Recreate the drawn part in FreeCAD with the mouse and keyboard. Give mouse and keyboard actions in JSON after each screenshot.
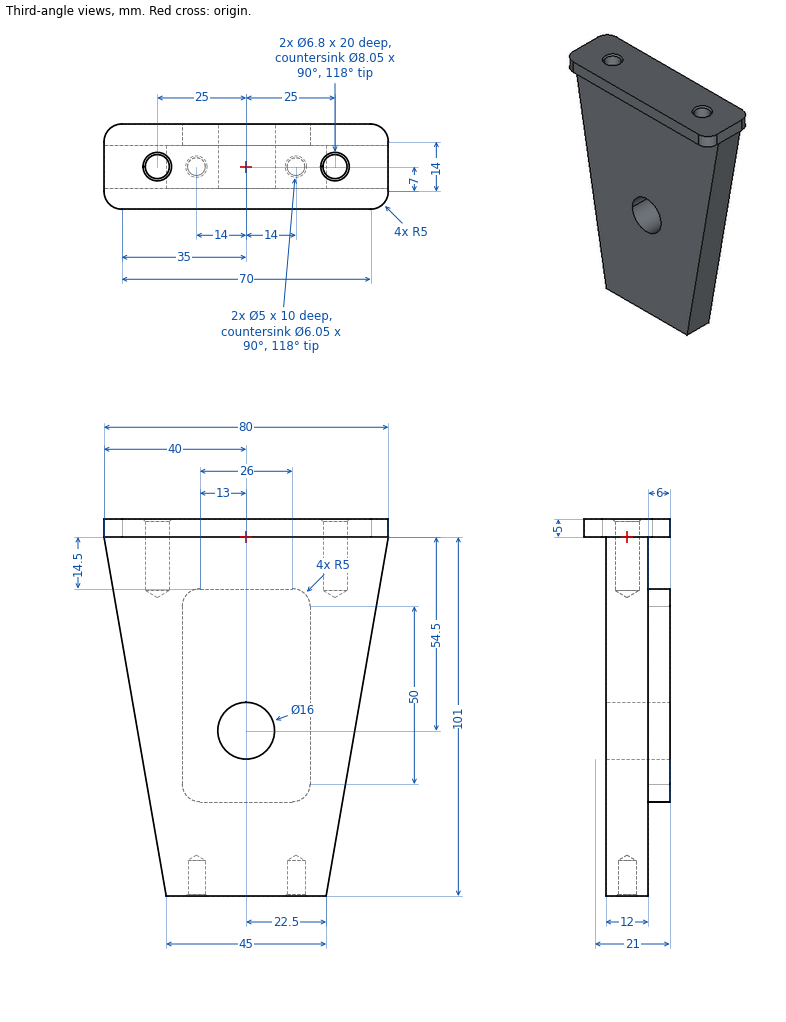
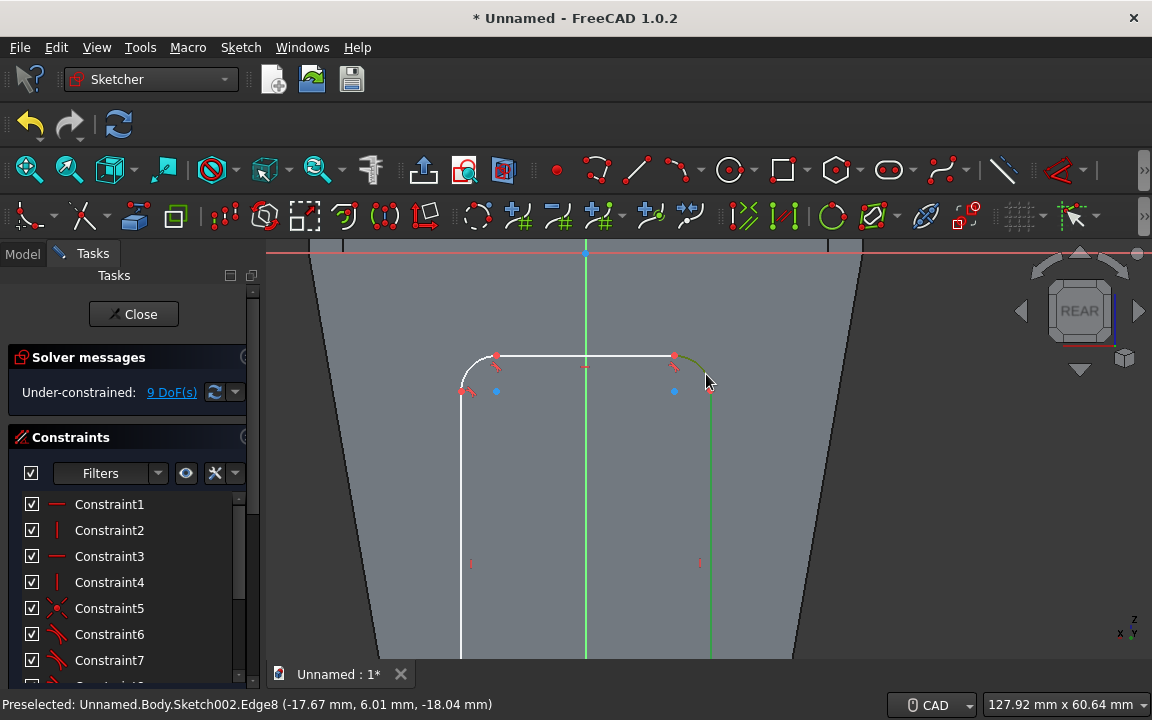
{"action": "key", "text": "t"}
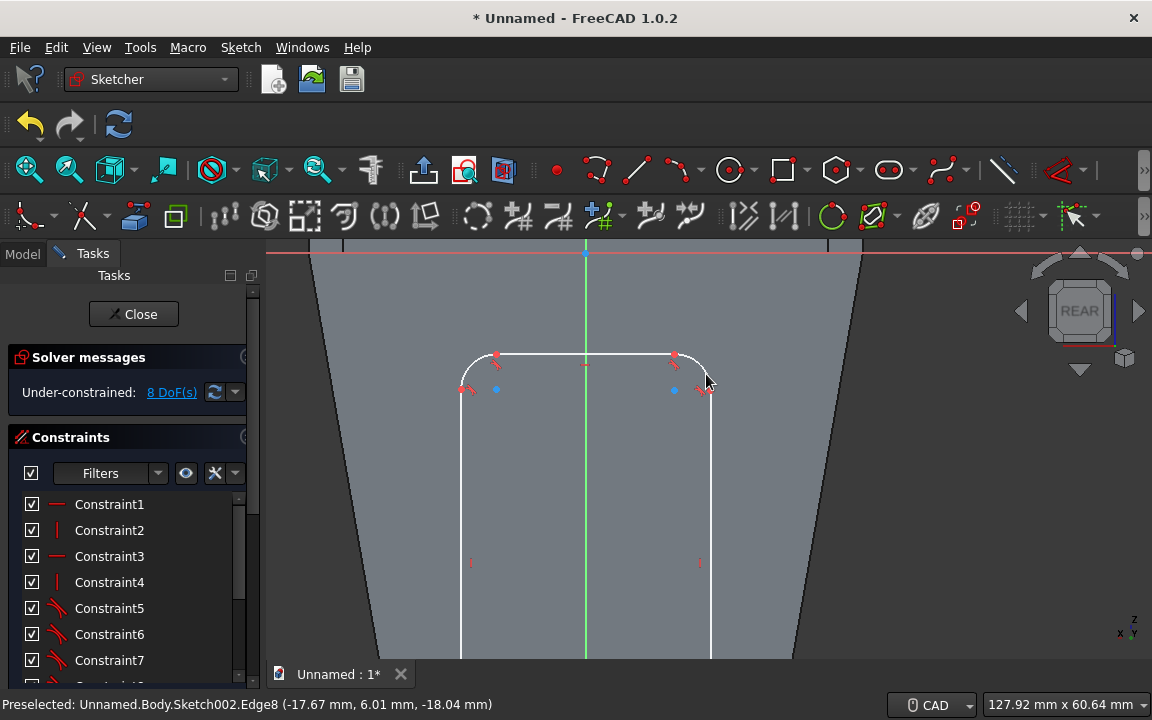
{"action": "left_click", "coordinate": [481, 358]}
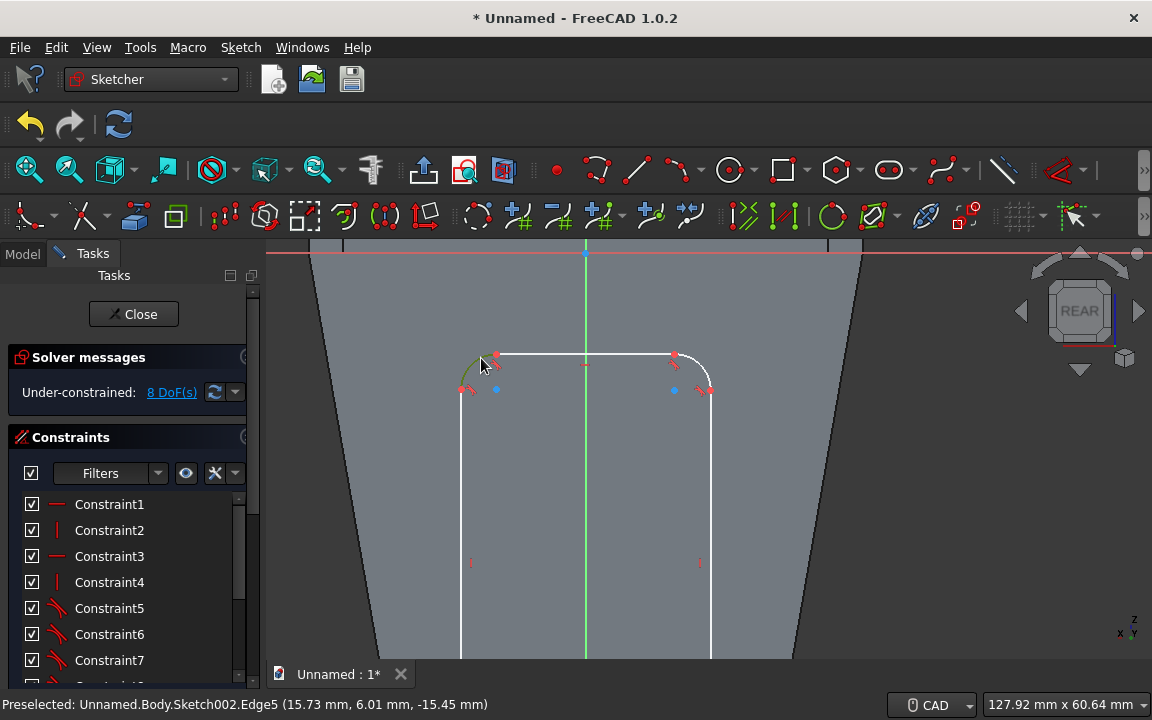
{"action": "scroll", "coordinate": [707, 373], "scroll_direction": "down", "scroll_amount": 3}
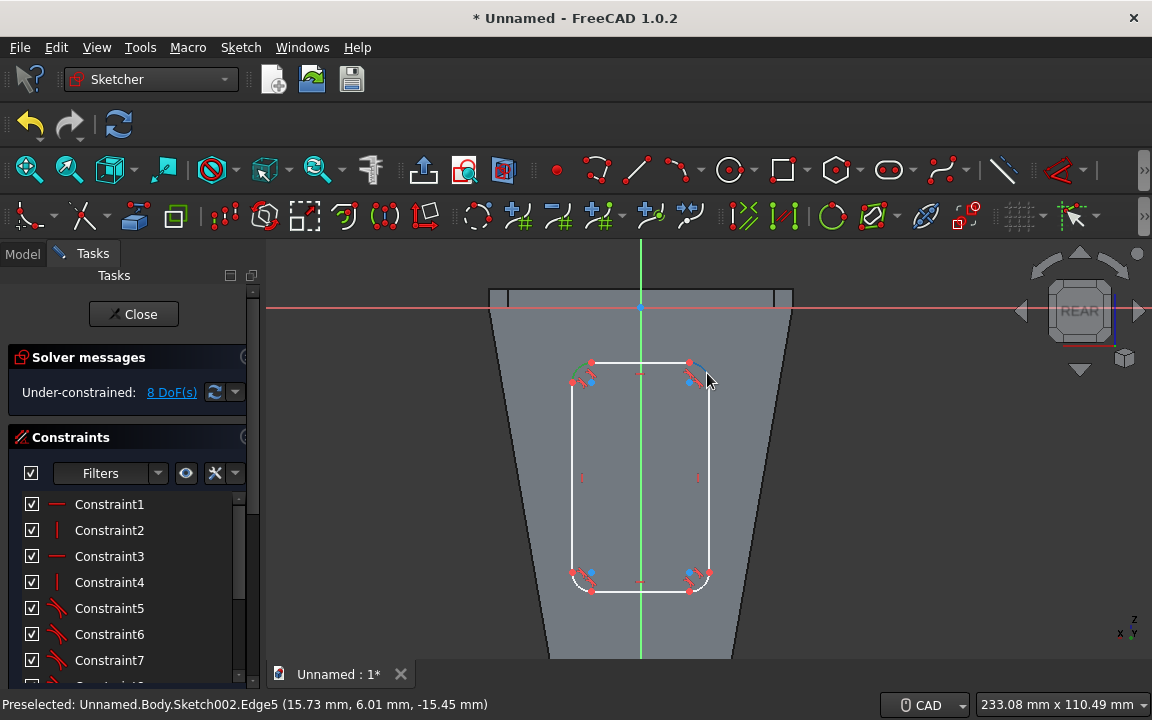
{"action": "scroll", "coordinate": [574, 581], "scroll_direction": "up", "scroll_amount": 3}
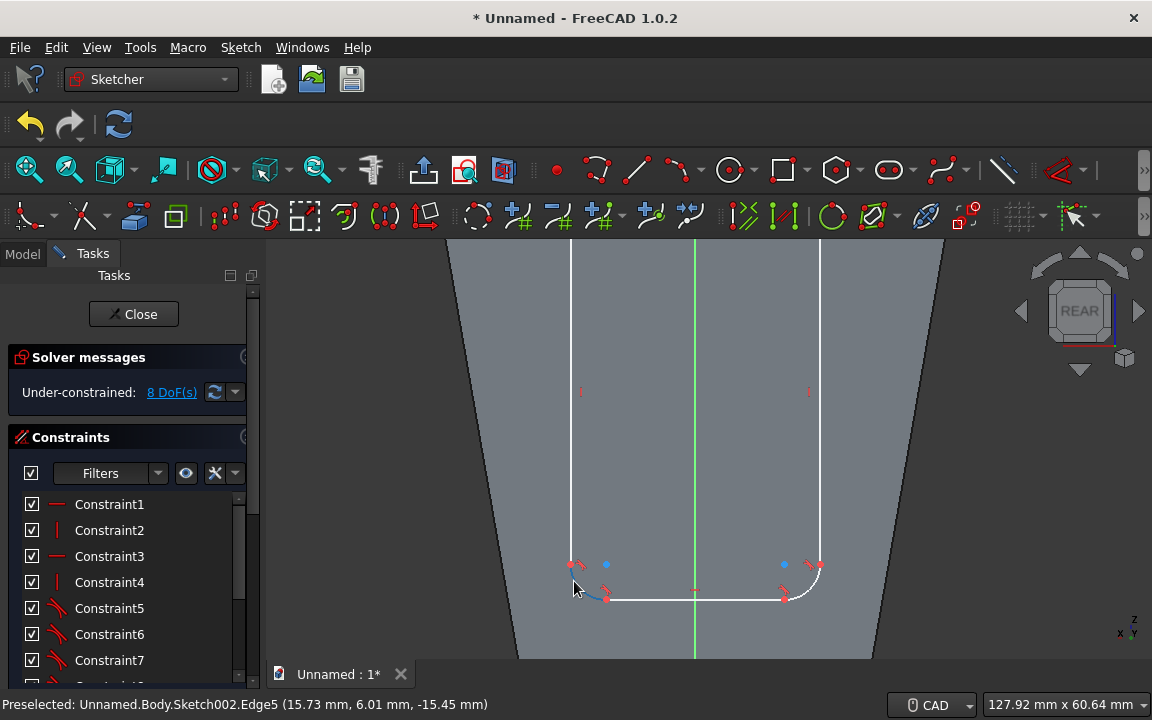
{"action": "left_click", "coordinate": [574, 580]}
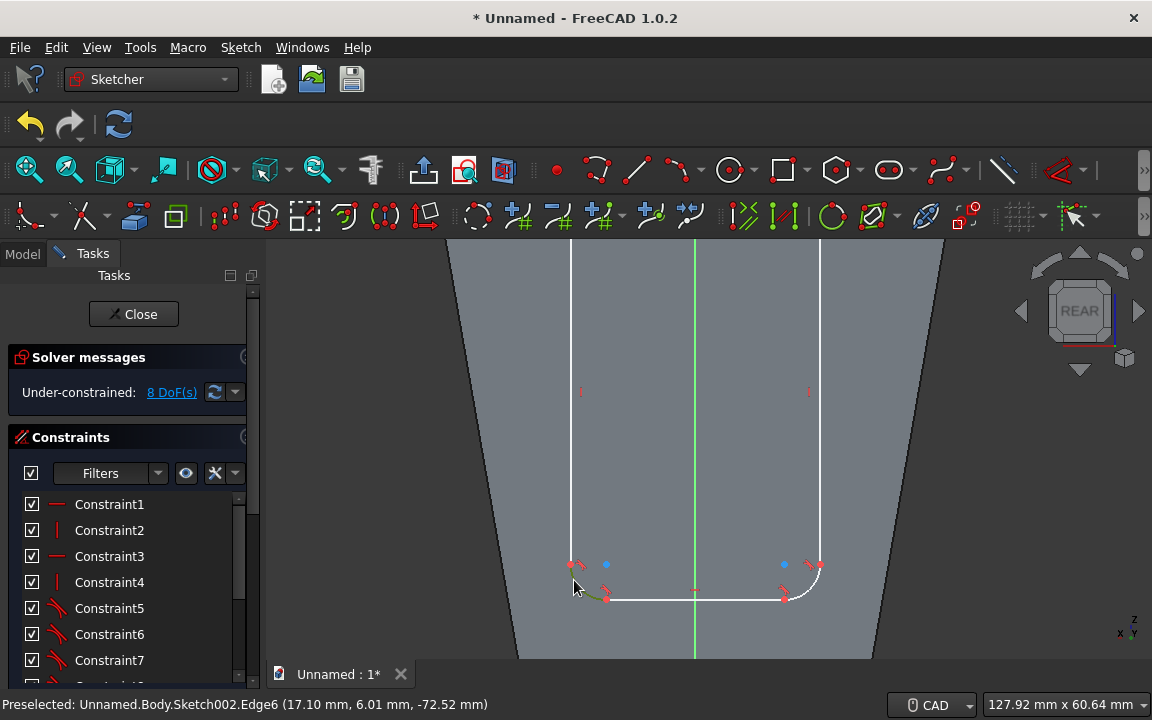
{"action": "left_click", "coordinate": [801, 596]}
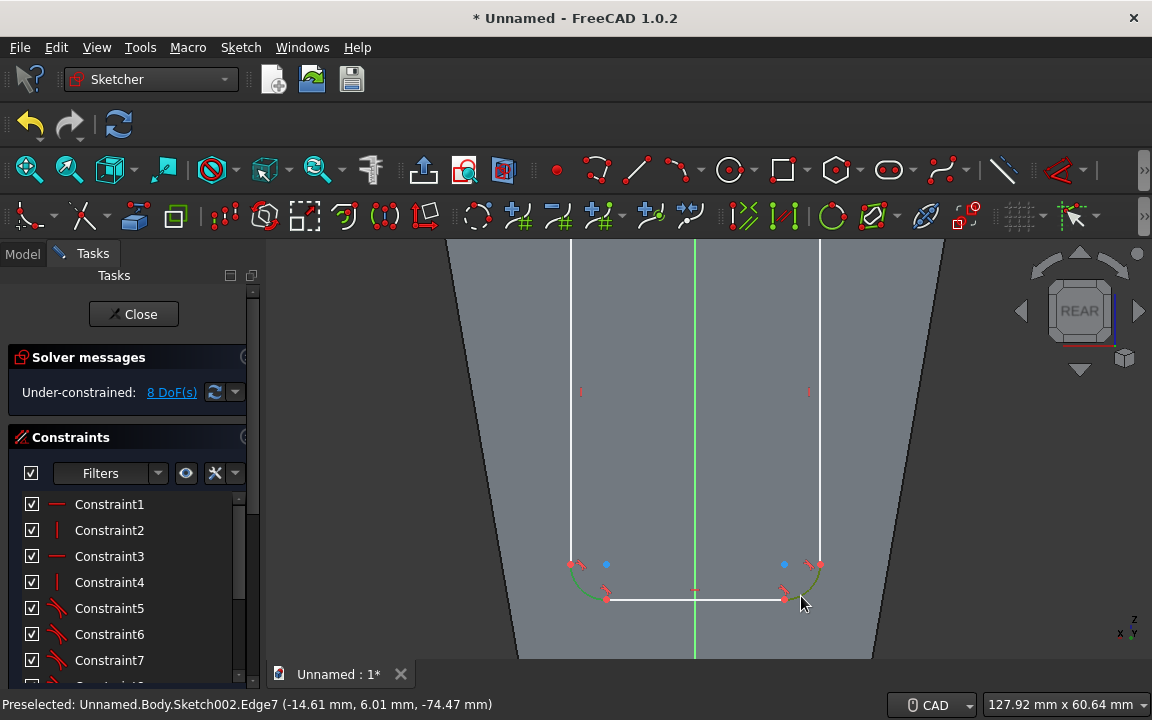
{"action": "scroll", "coordinate": [574, 582], "scroll_direction": "down", "scroll_amount": 3}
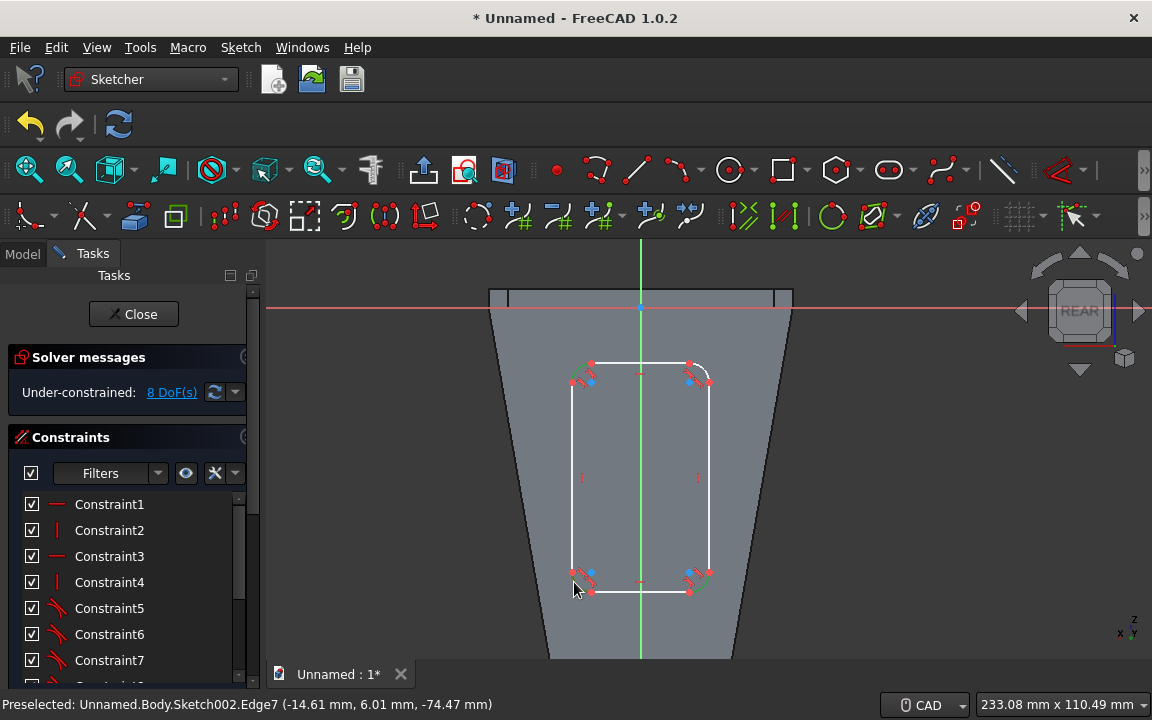
{"action": "scroll", "coordinate": [707, 374], "scroll_direction": "up", "scroll_amount": 3}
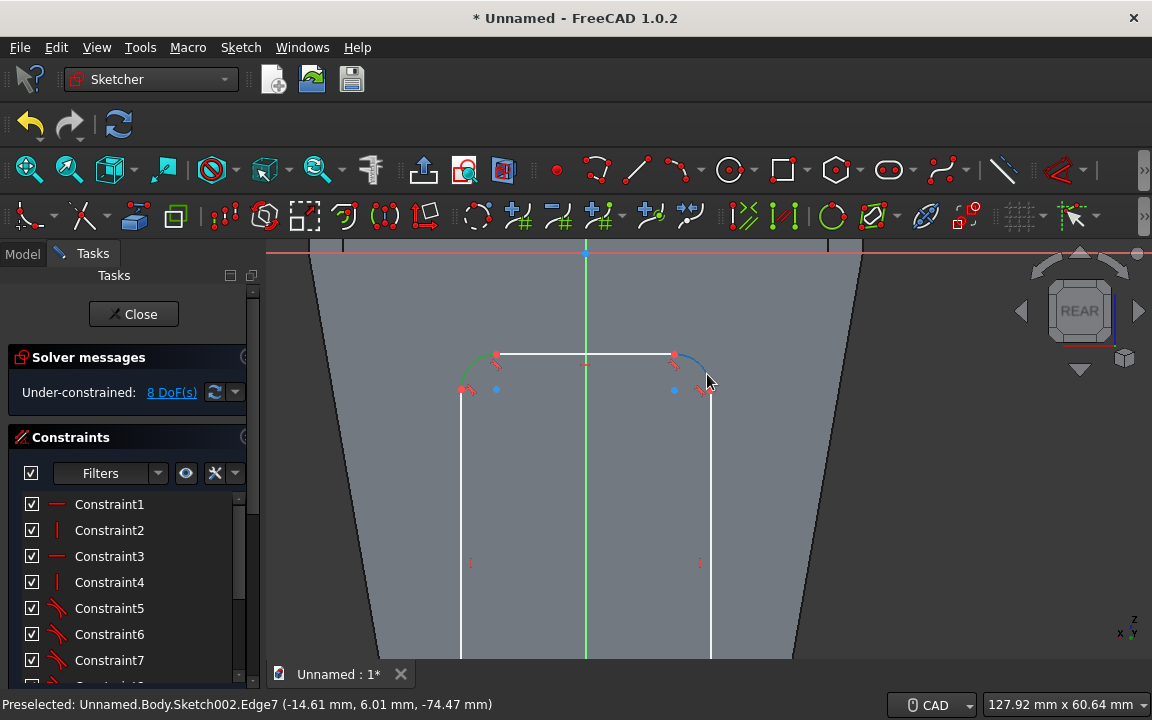
{"action": "left_click", "coordinate": [707, 374]}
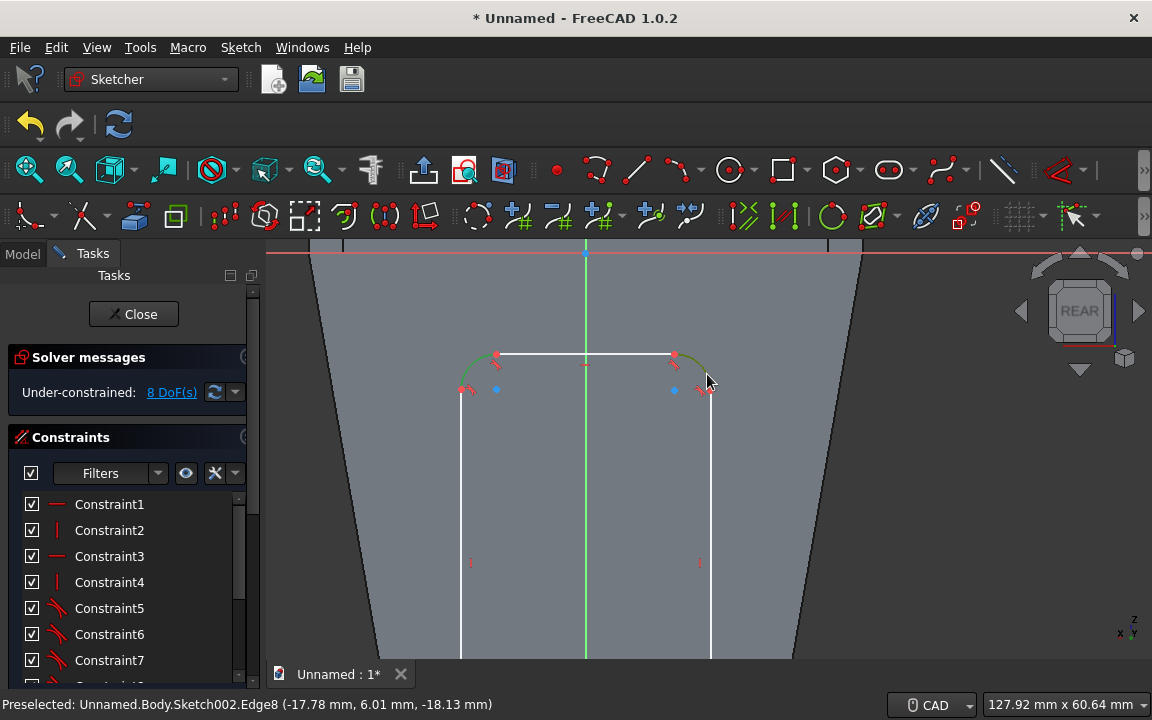
{"action": "key", "text": "e"}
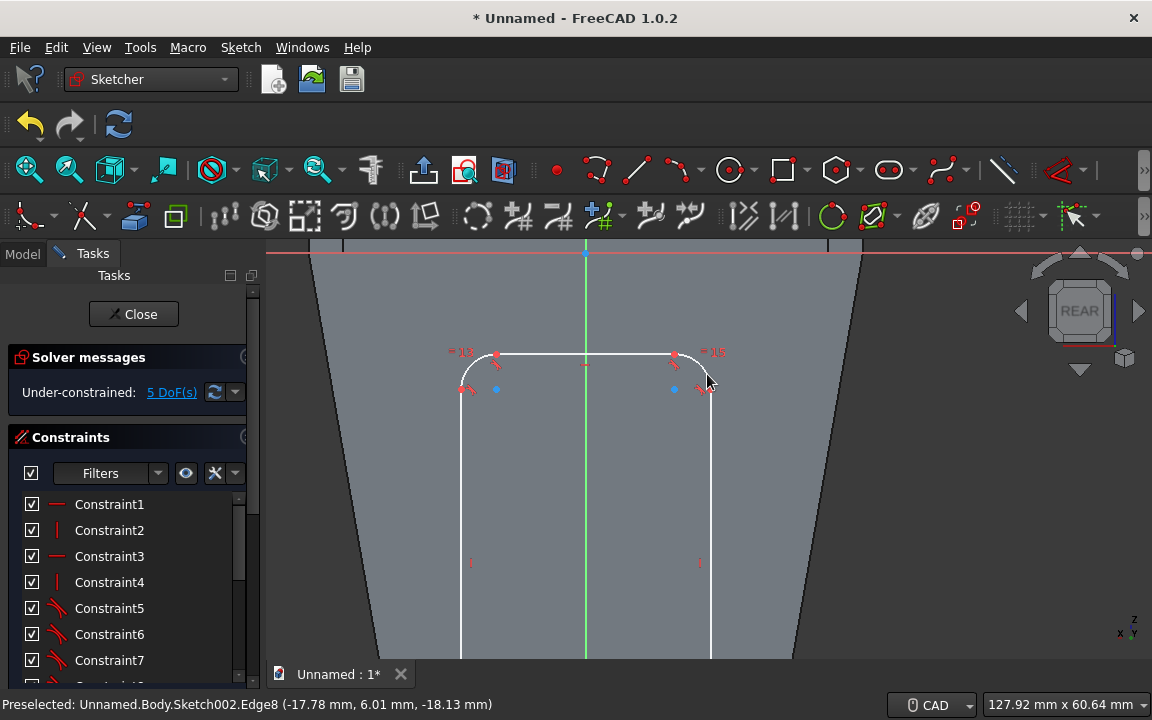
{"action": "left_click", "coordinate": [1058, 170]}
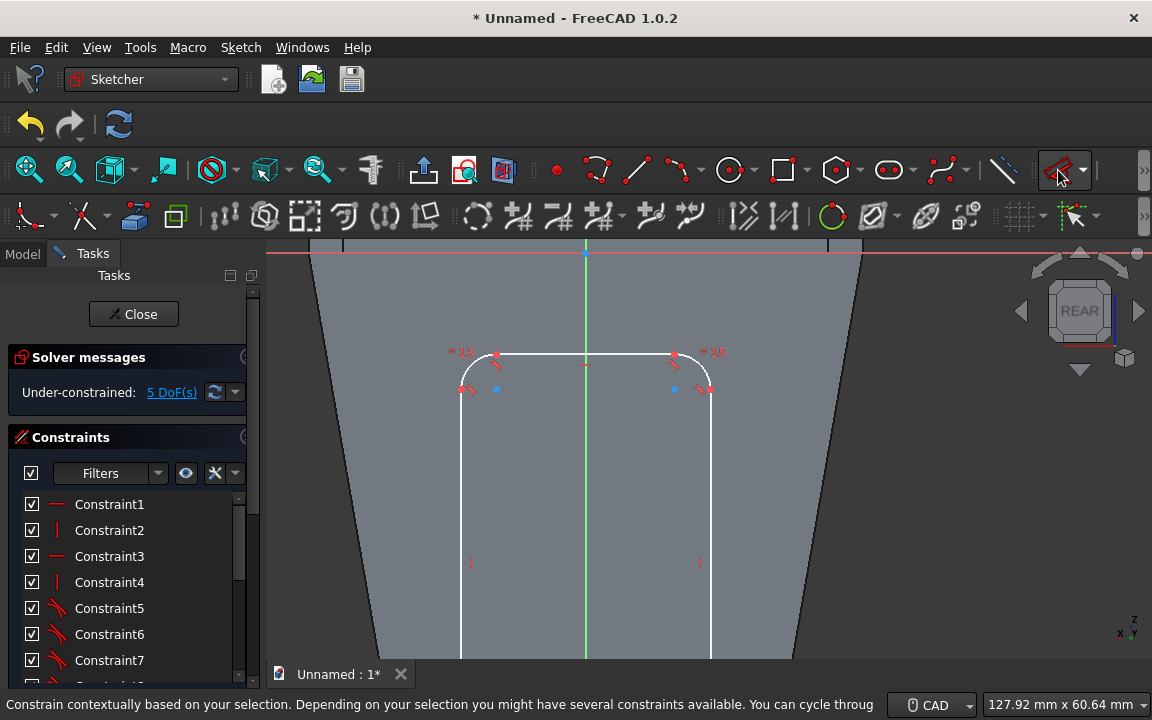
{"action": "left_click", "coordinate": [481, 358]}
{"action": "left_click", "coordinate": [467, 329]}